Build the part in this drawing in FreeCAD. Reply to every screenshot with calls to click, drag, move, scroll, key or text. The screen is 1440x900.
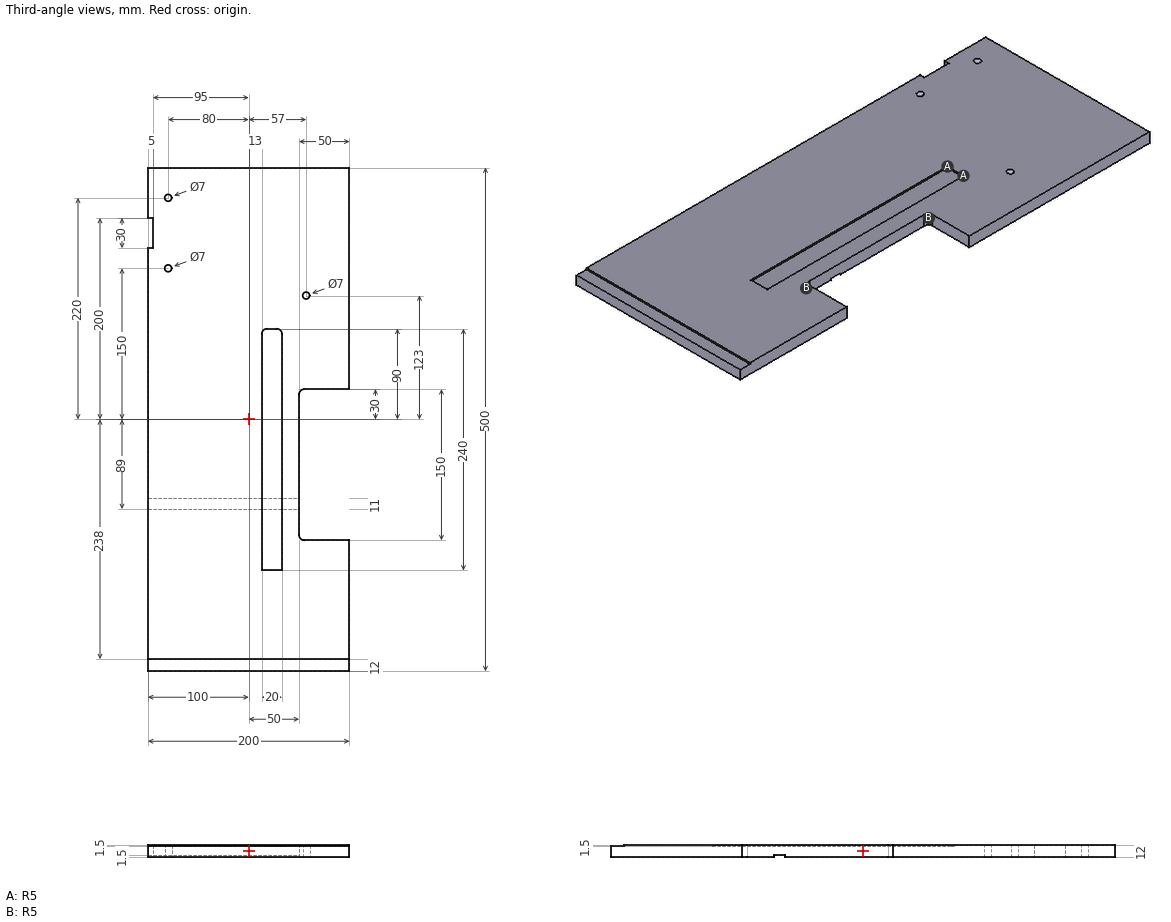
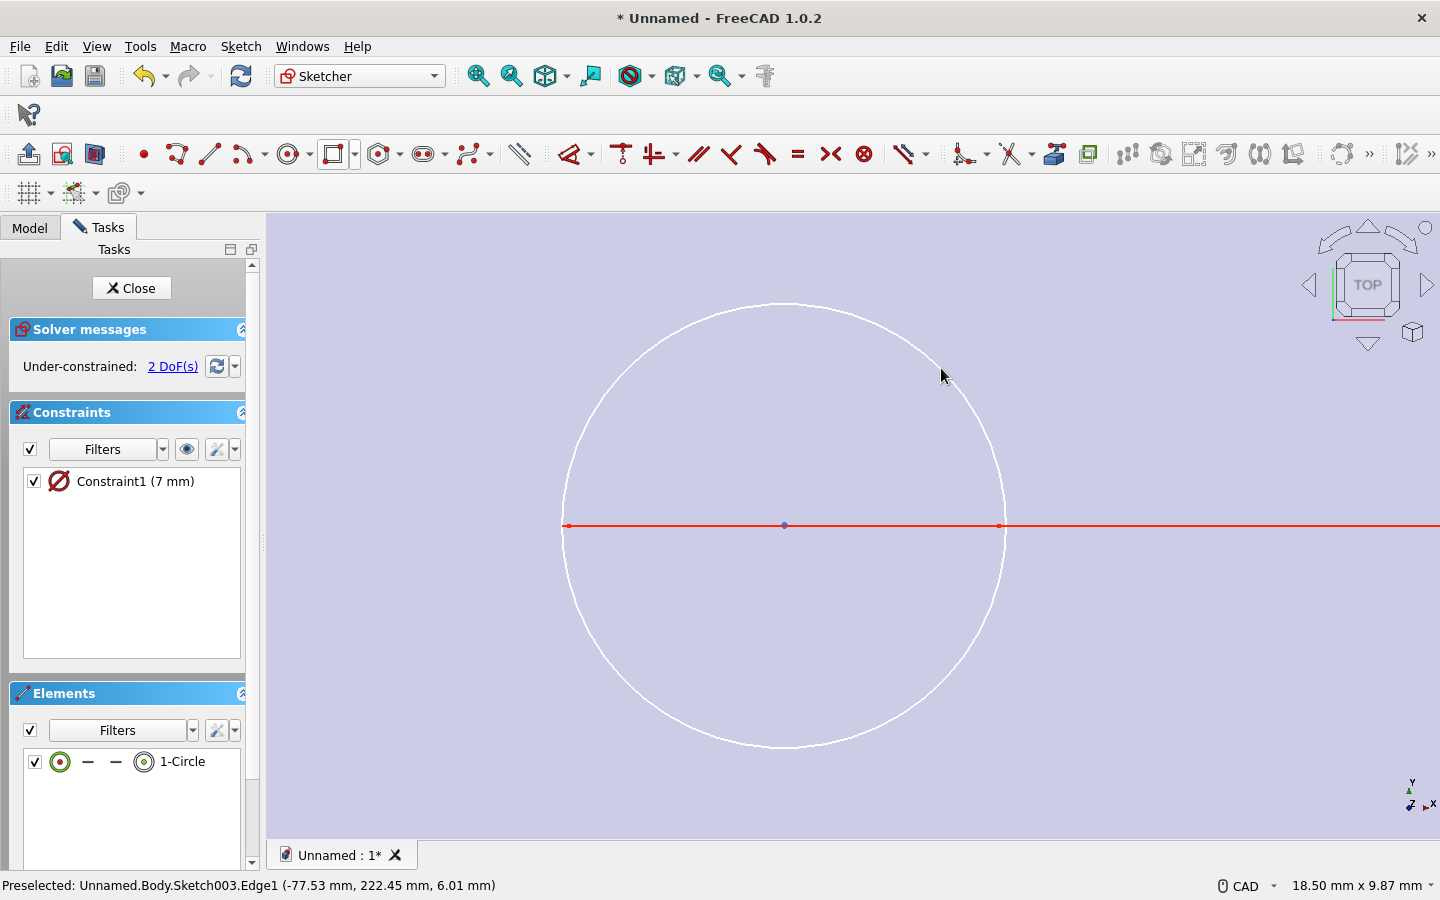
key(d)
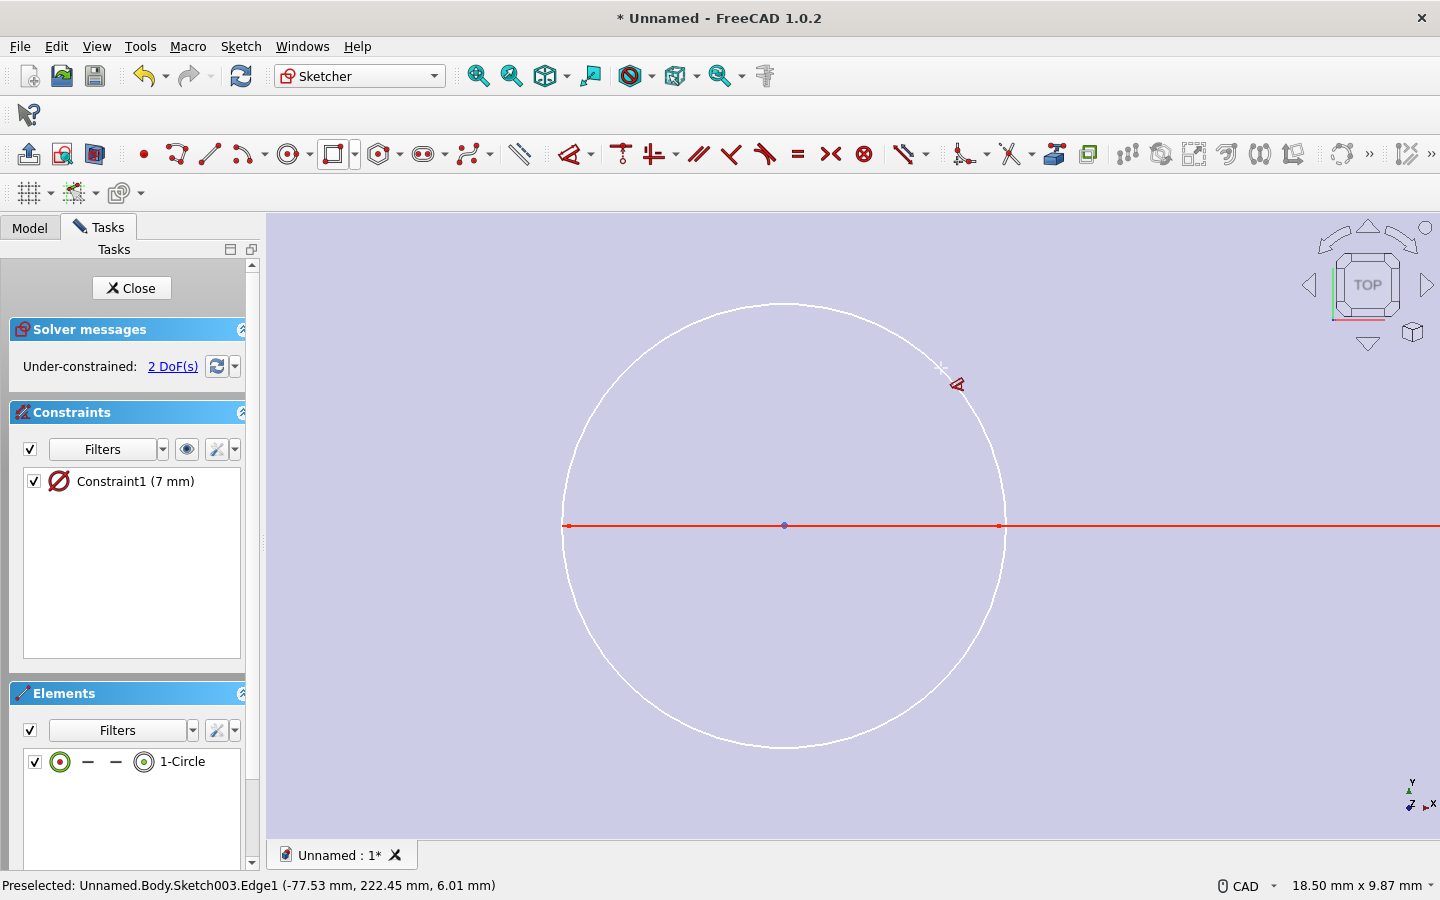
click(784, 526)
click(1030, 492)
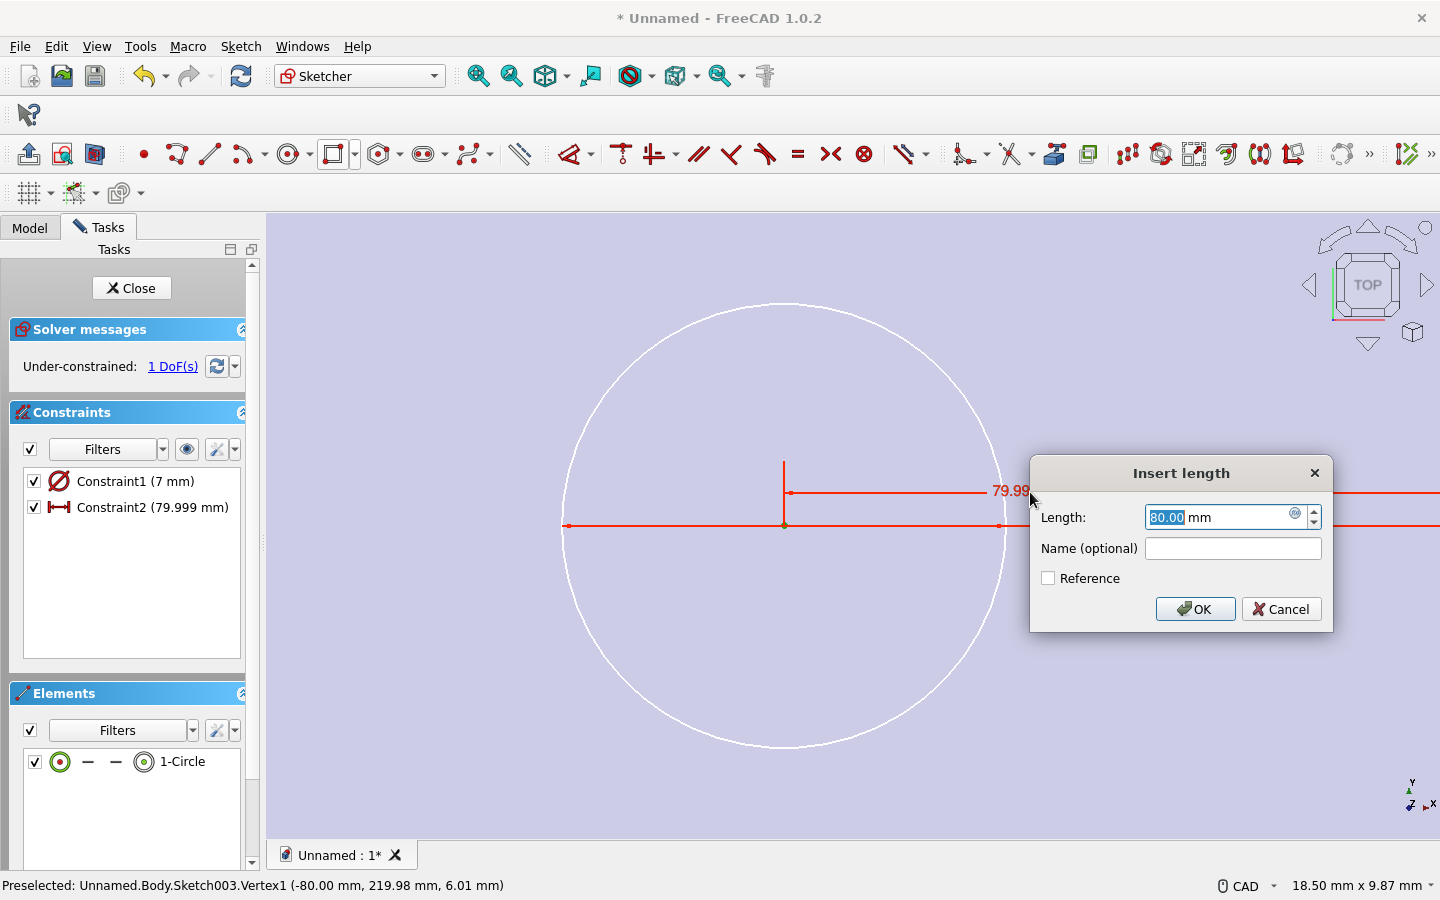
text(80)
key(Return)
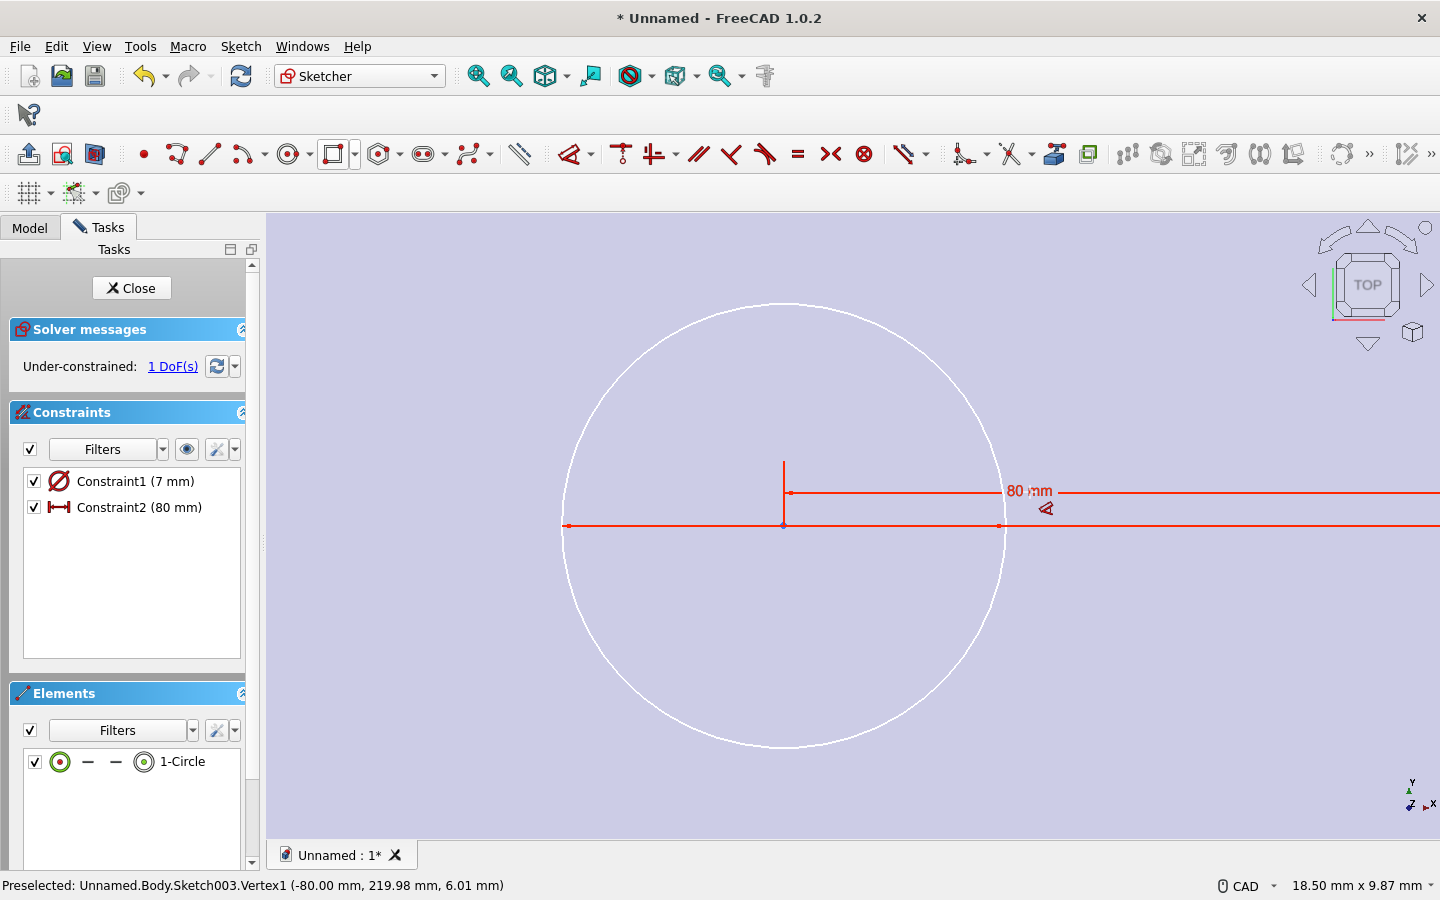
click(784, 526)
click(750, 668)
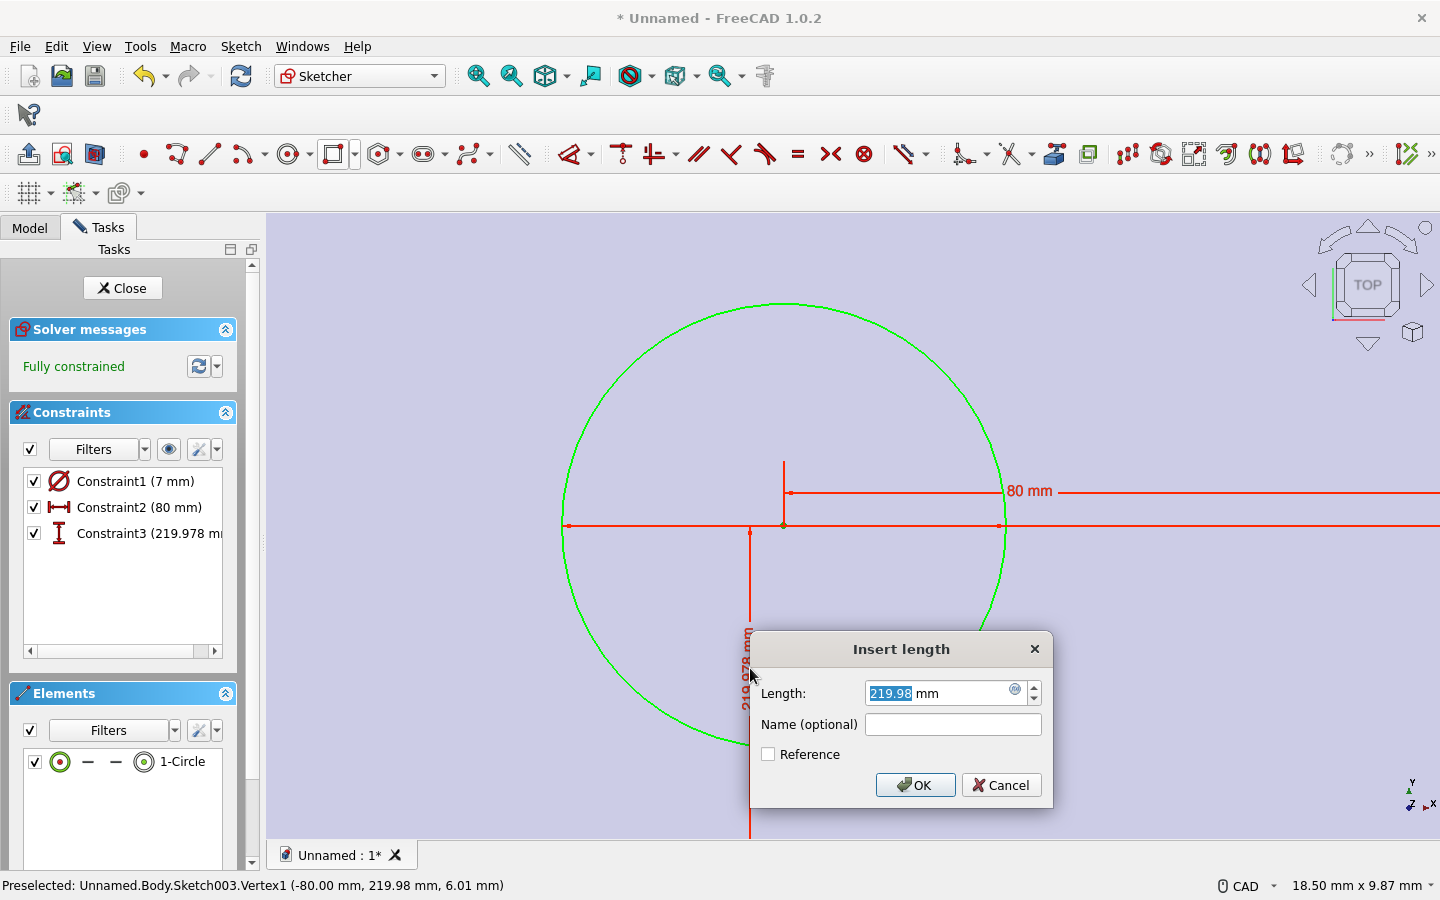
text(220)
key(Return)
key(Escape)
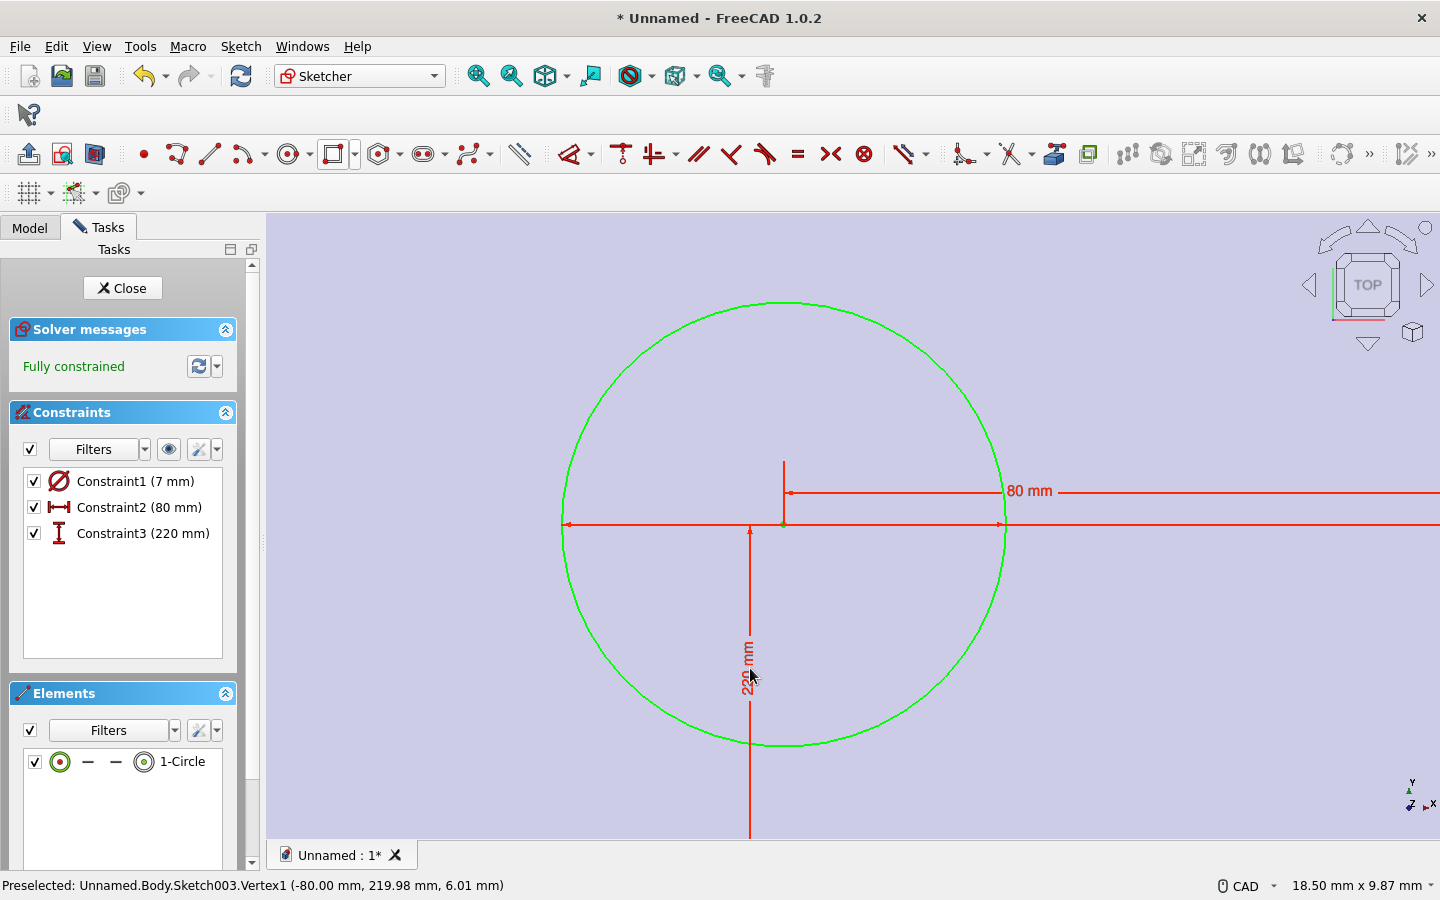
click(123, 288)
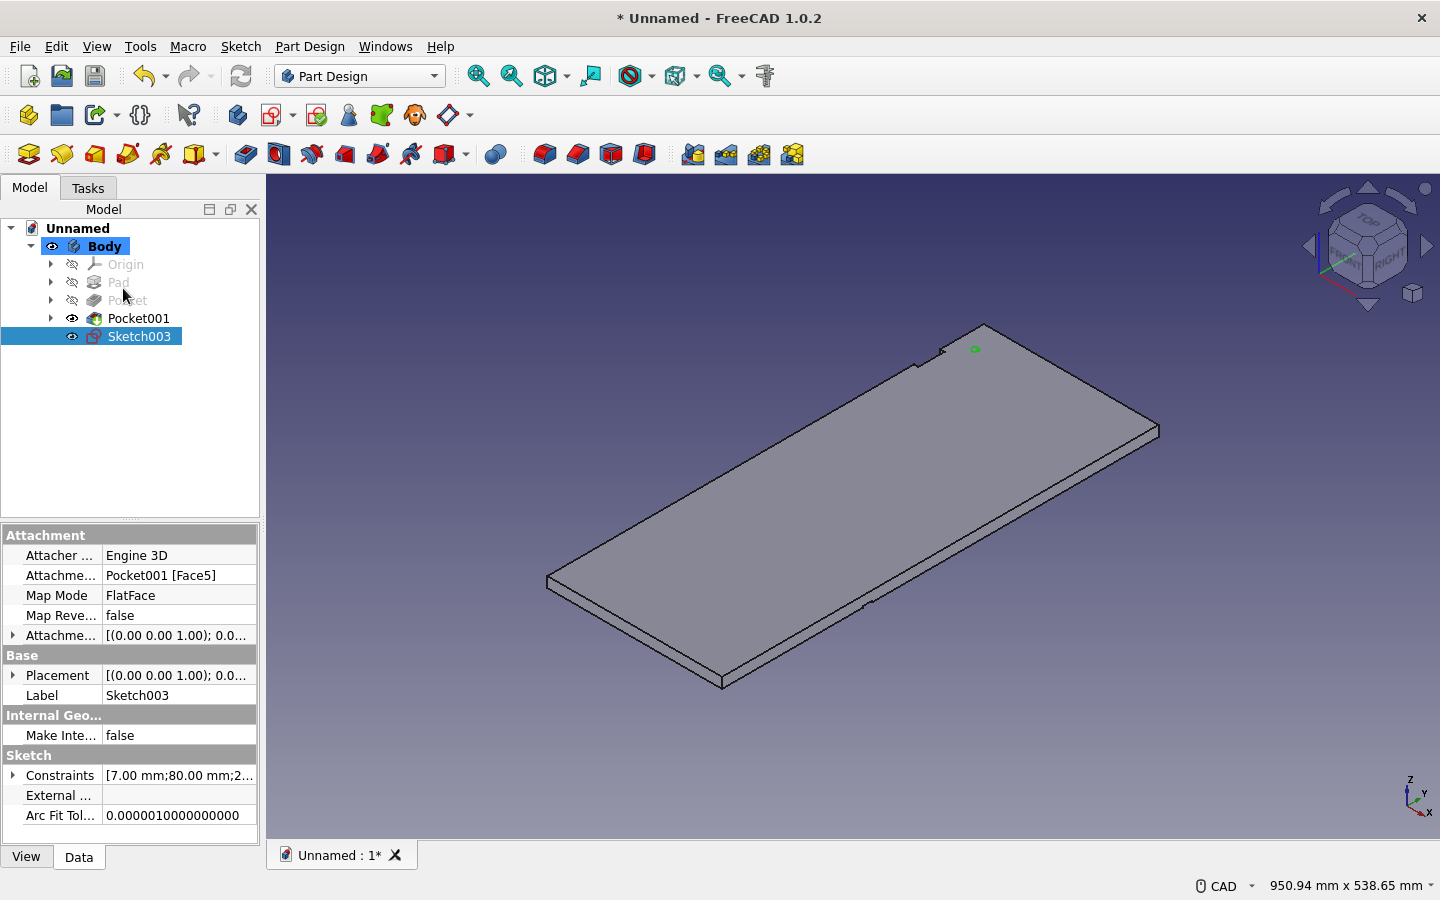
click(246, 154)